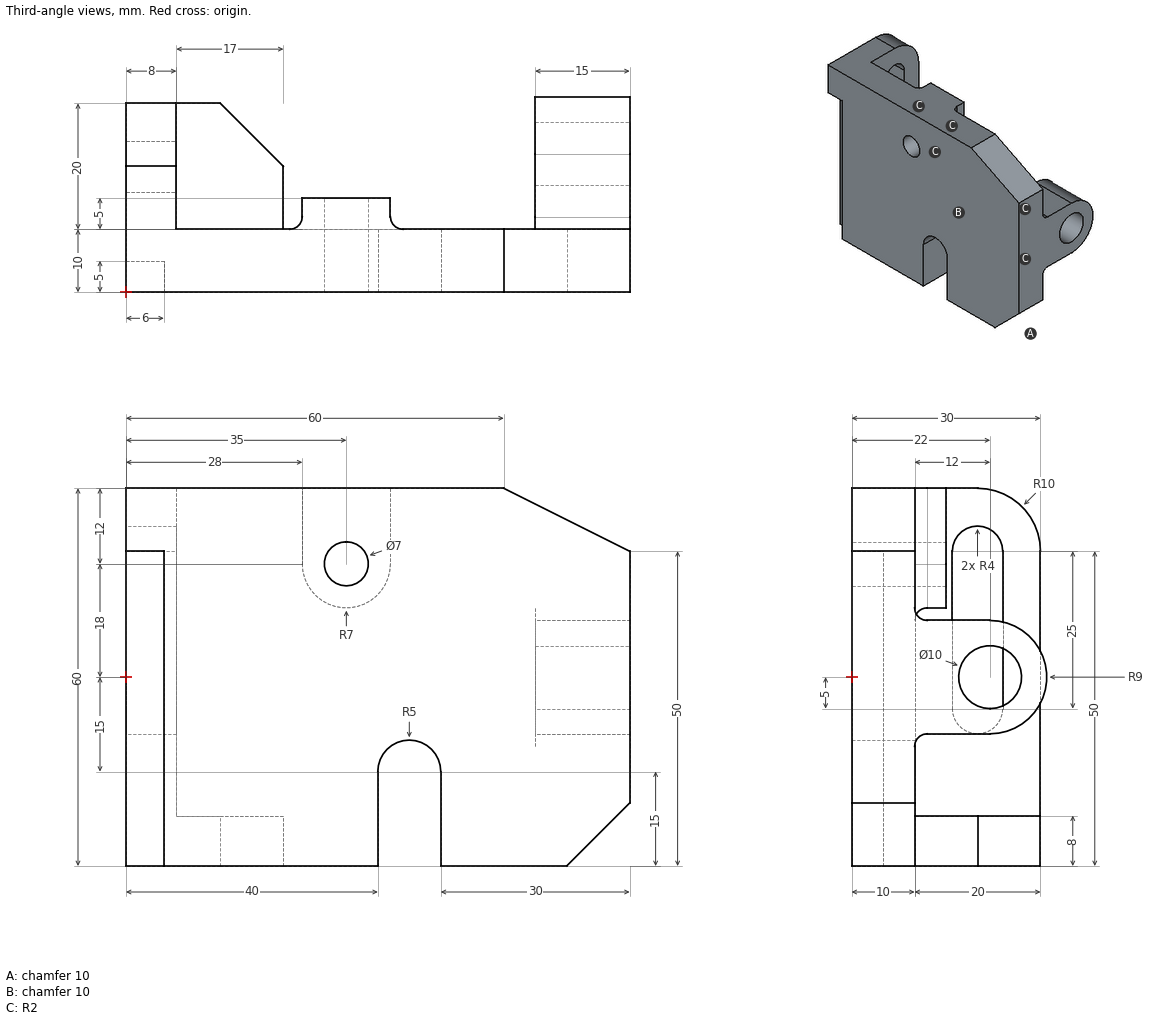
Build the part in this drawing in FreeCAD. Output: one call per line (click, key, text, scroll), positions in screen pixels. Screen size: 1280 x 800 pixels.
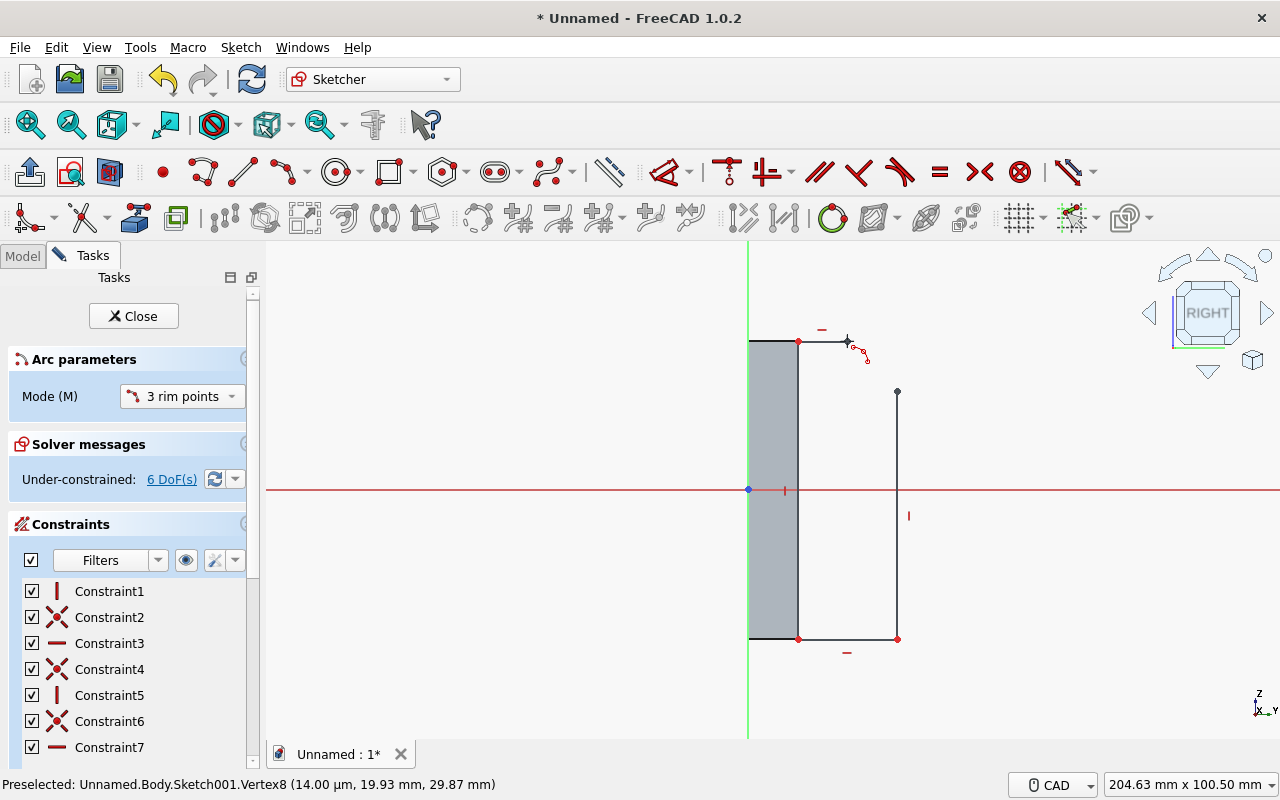
click(847, 342)
click(897, 392)
click(882, 356)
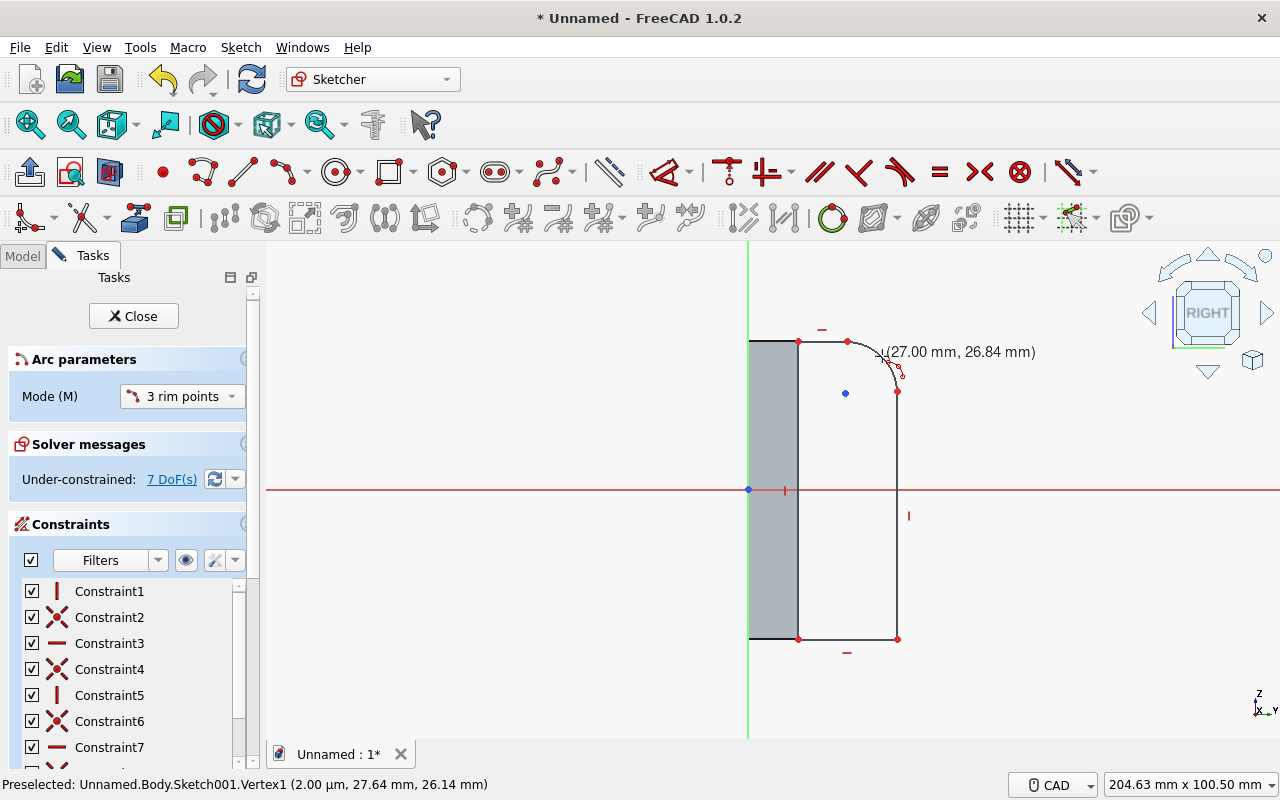
click(496, 172)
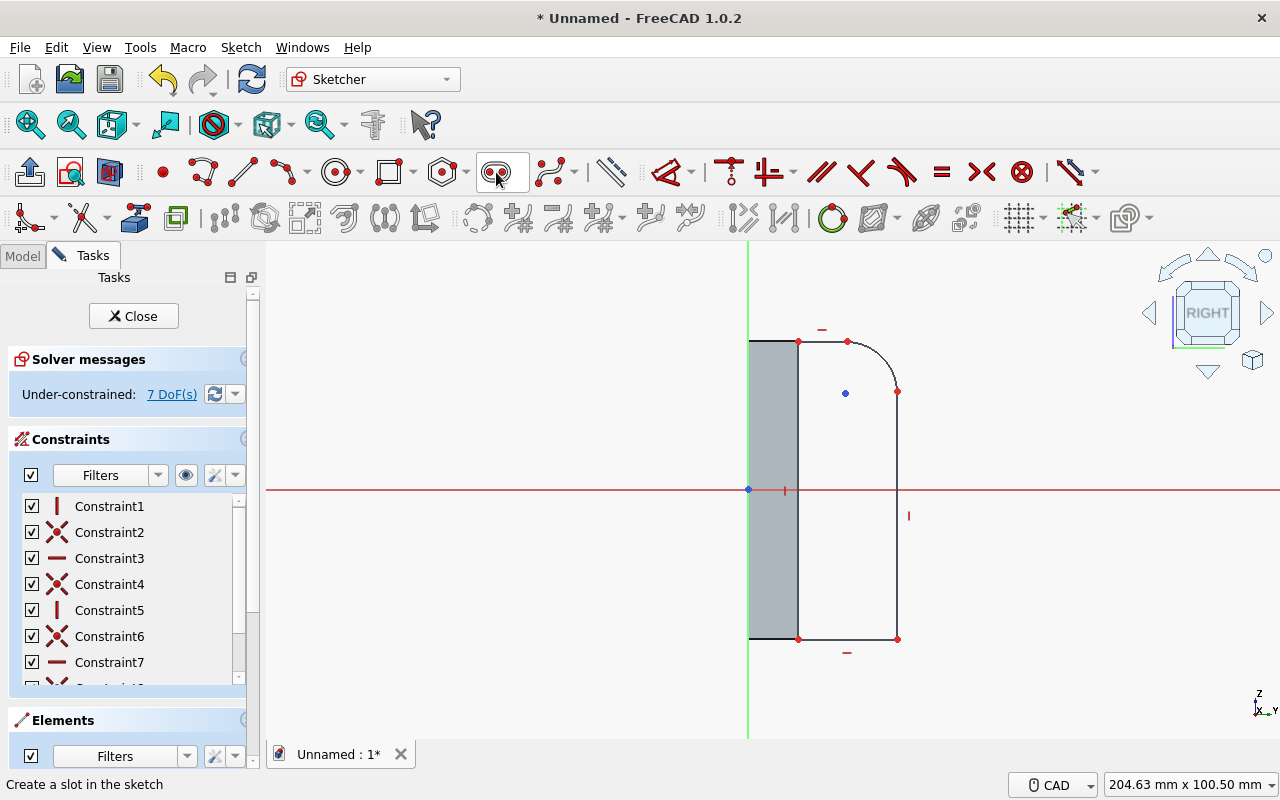
click(847, 515)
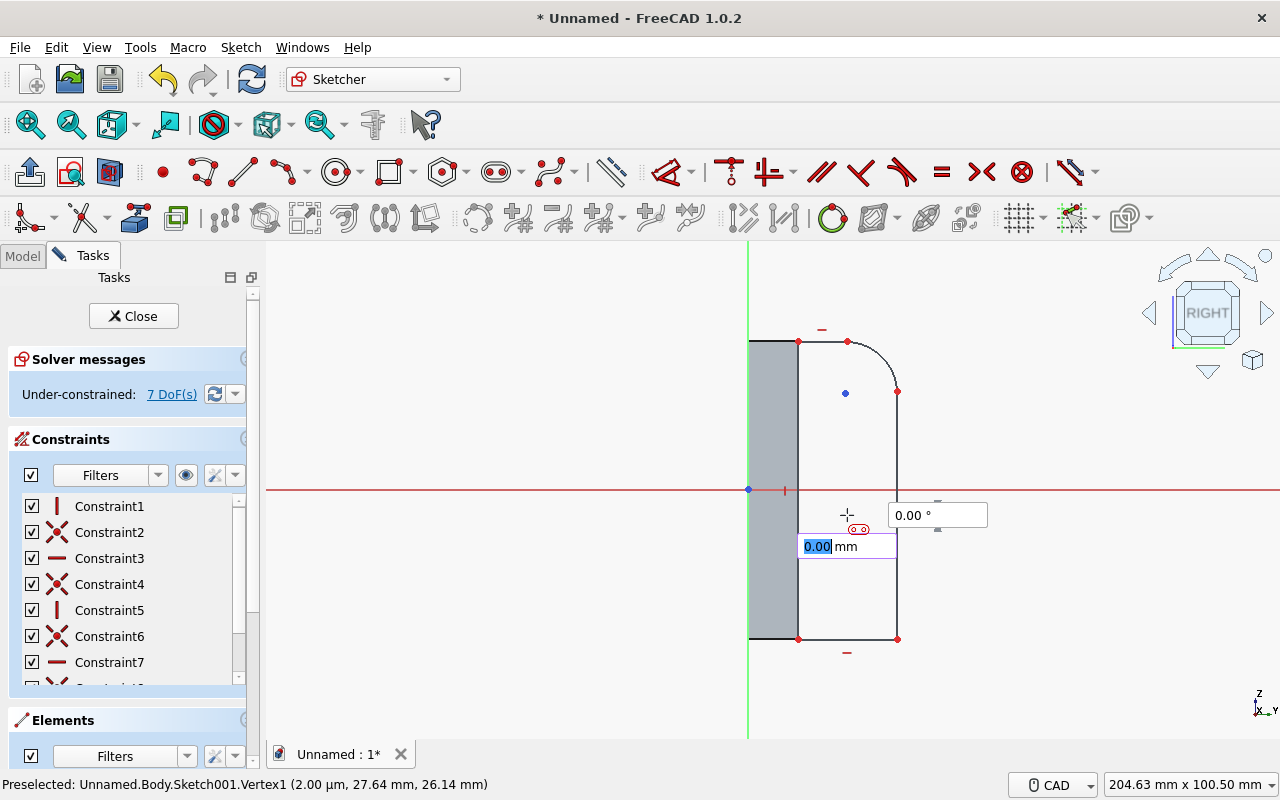
click(847, 391)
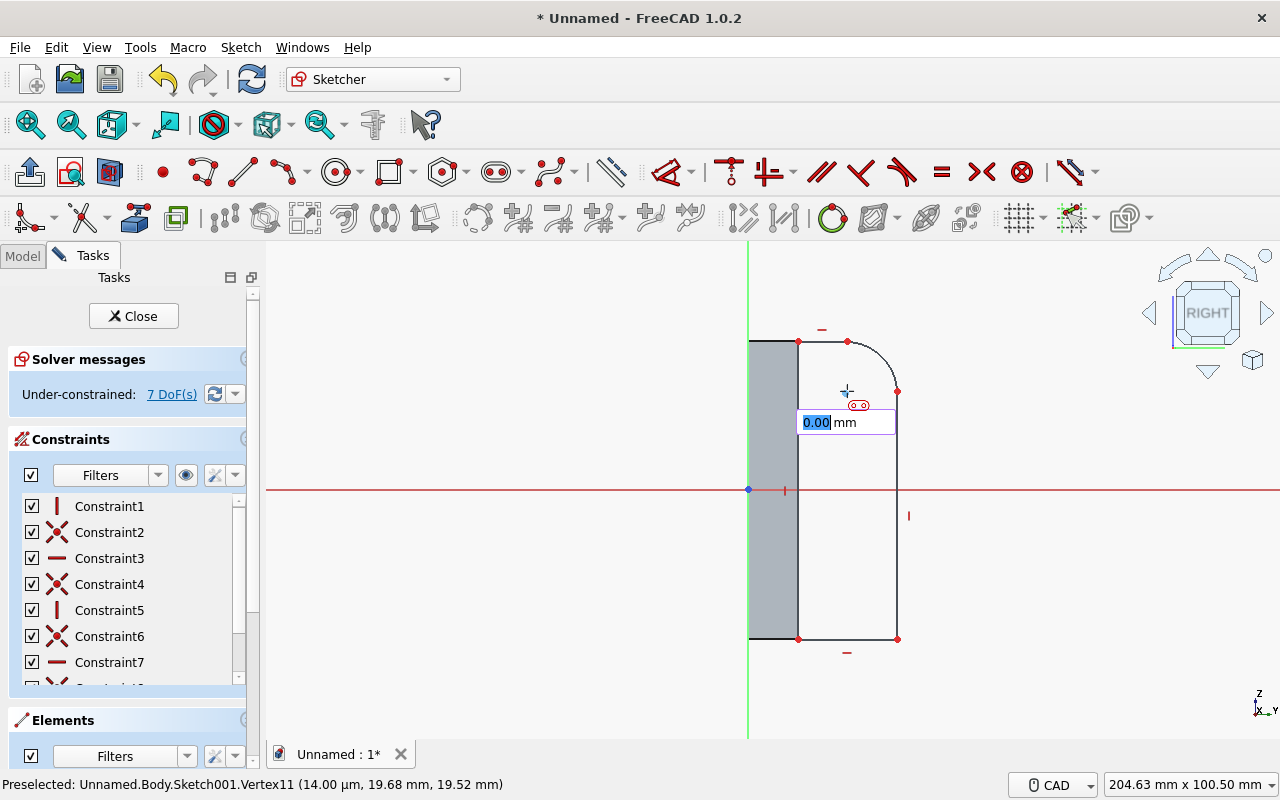
click(828, 453)
key(Escape)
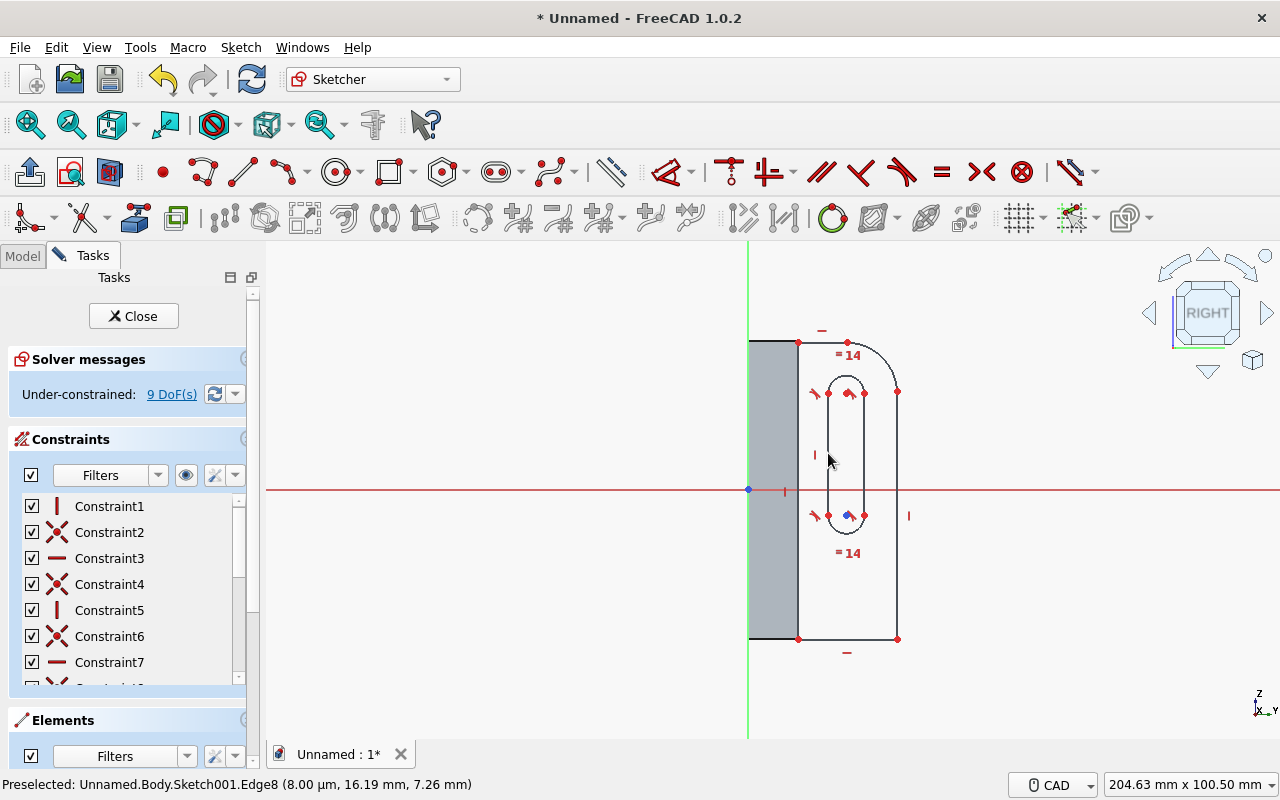
click(897, 466)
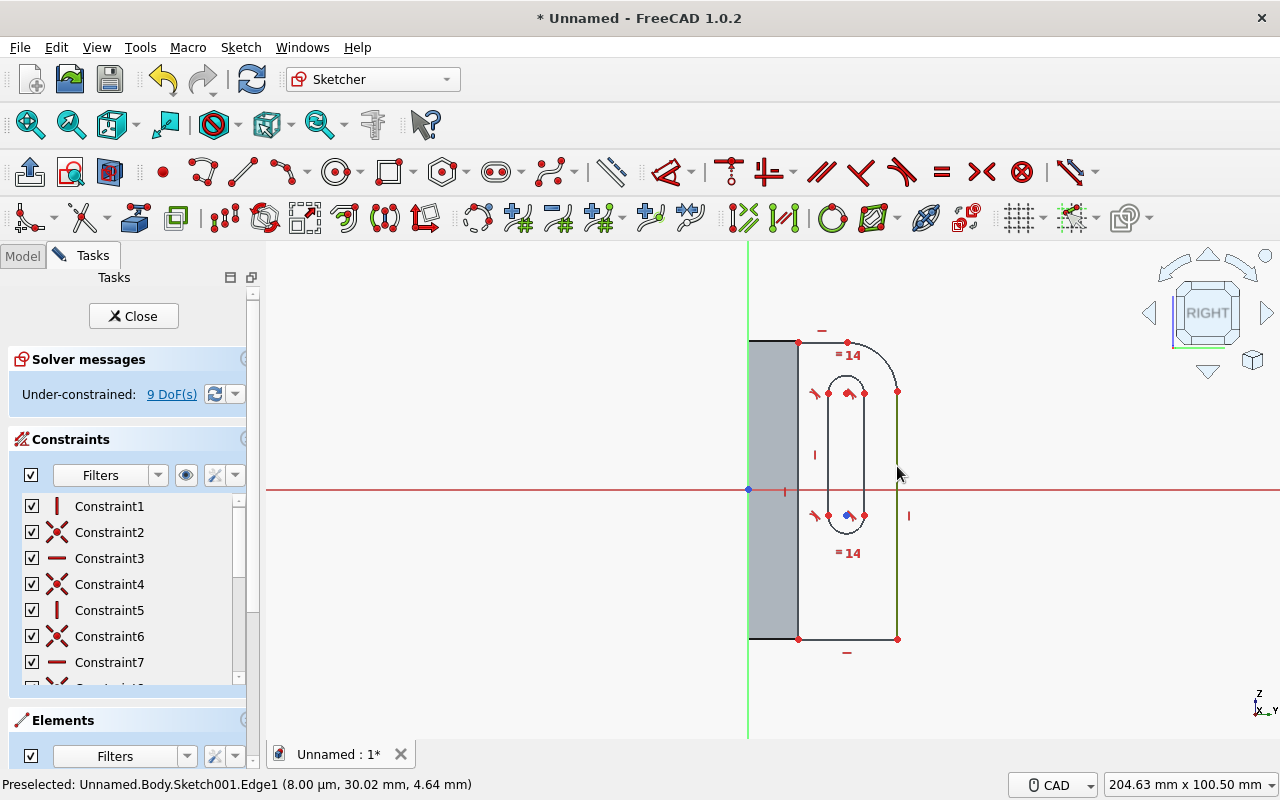
click(891, 370)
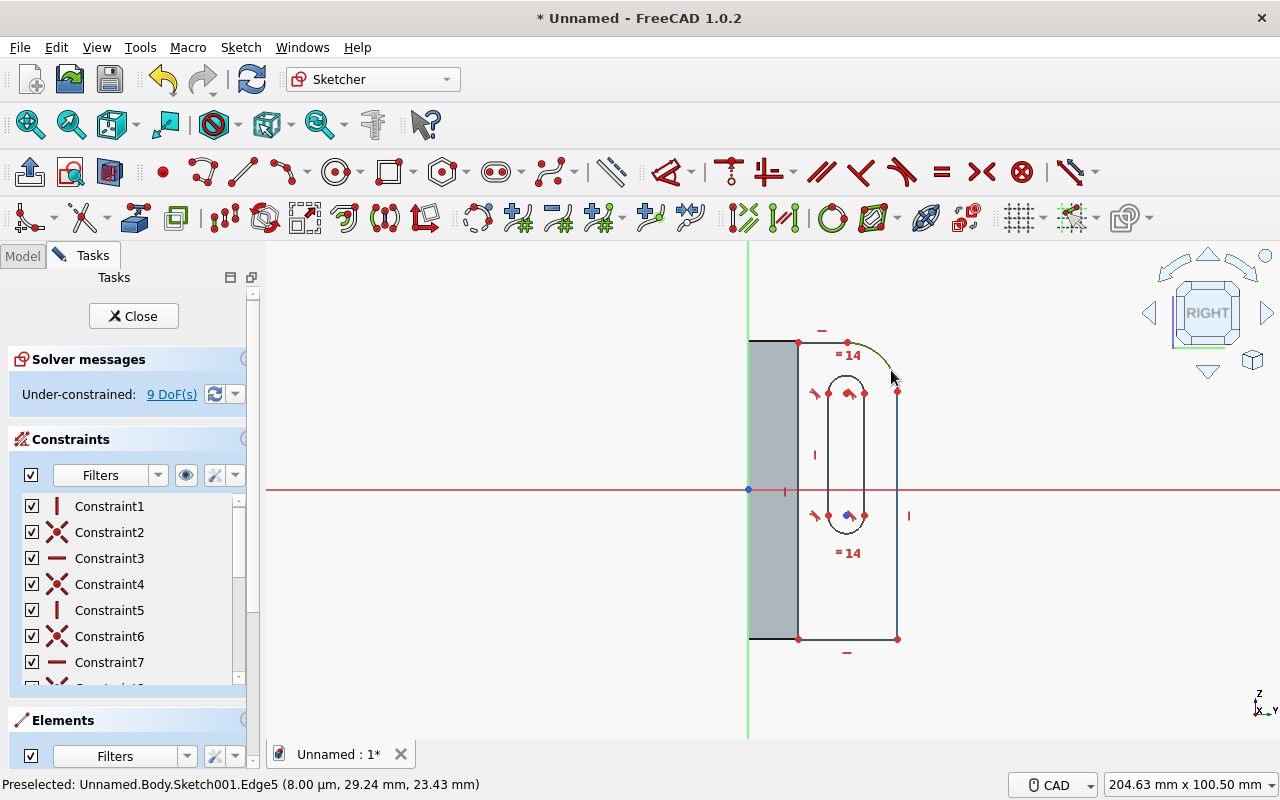
click(902, 172)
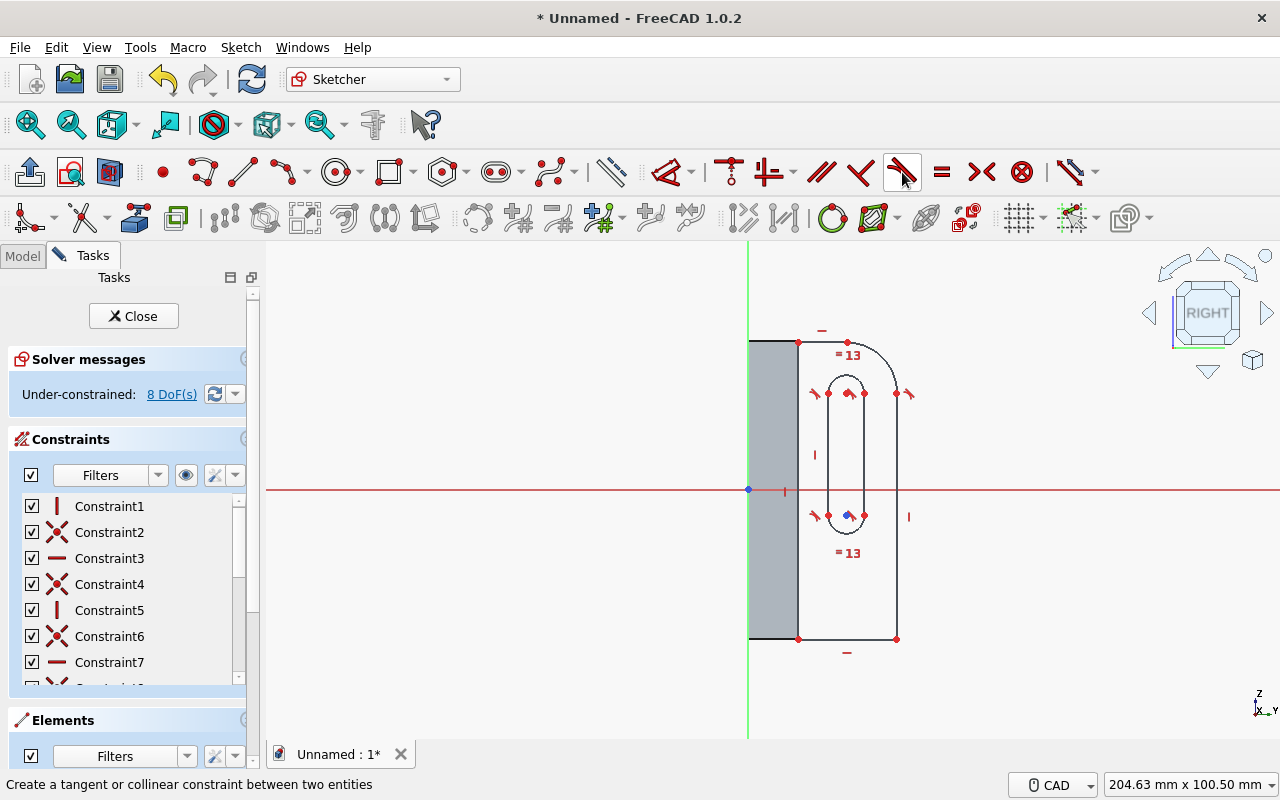
click(813, 342)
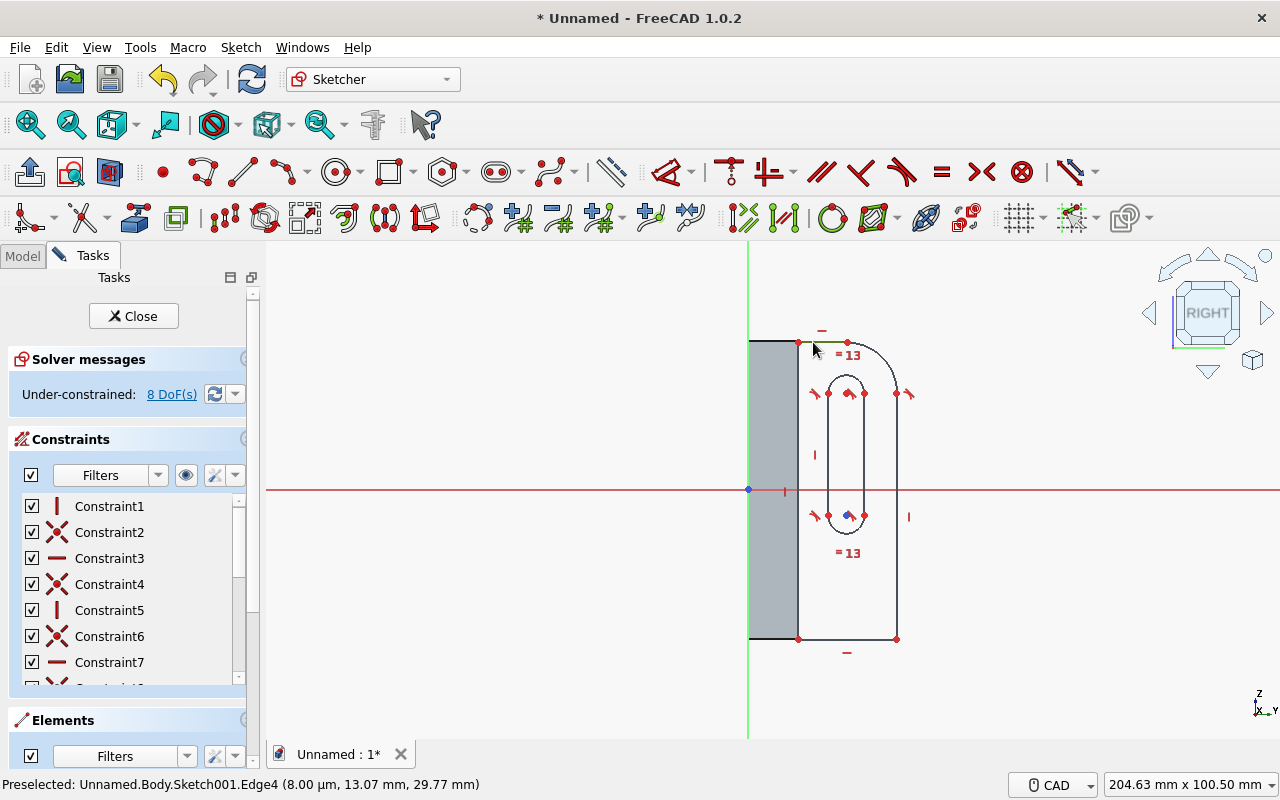
click(892, 370)